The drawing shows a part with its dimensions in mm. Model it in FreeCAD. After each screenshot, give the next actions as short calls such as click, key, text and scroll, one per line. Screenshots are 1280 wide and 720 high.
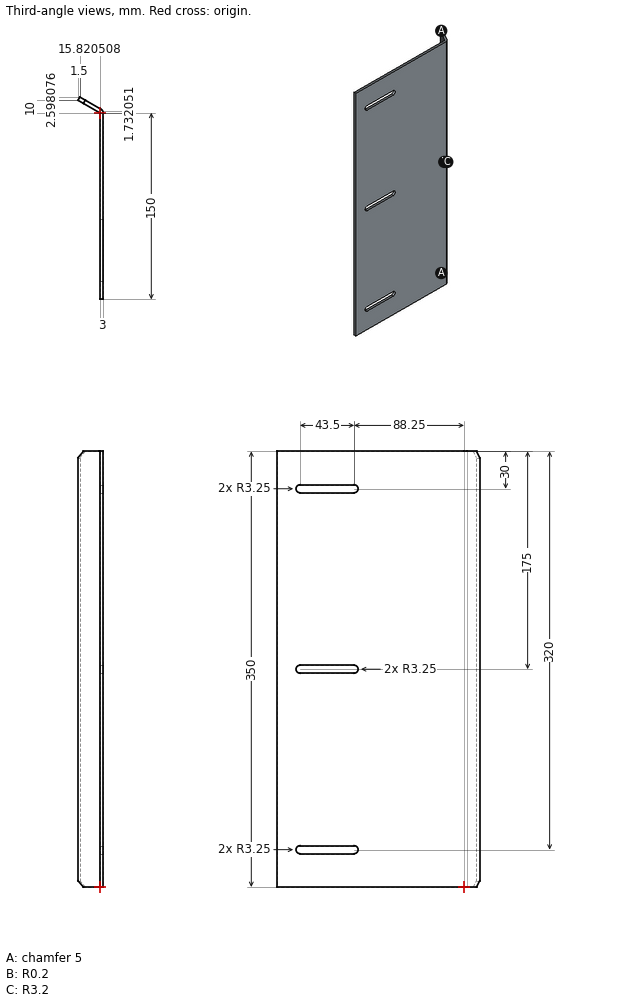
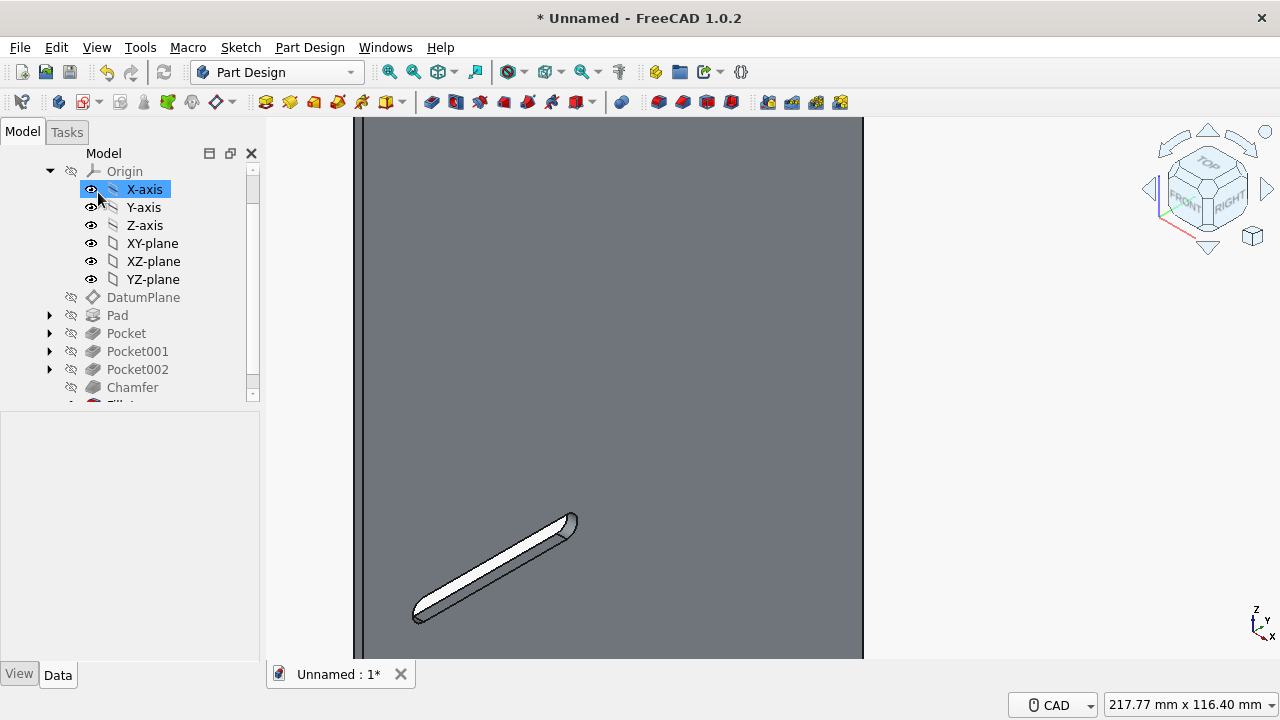
click(390, 72)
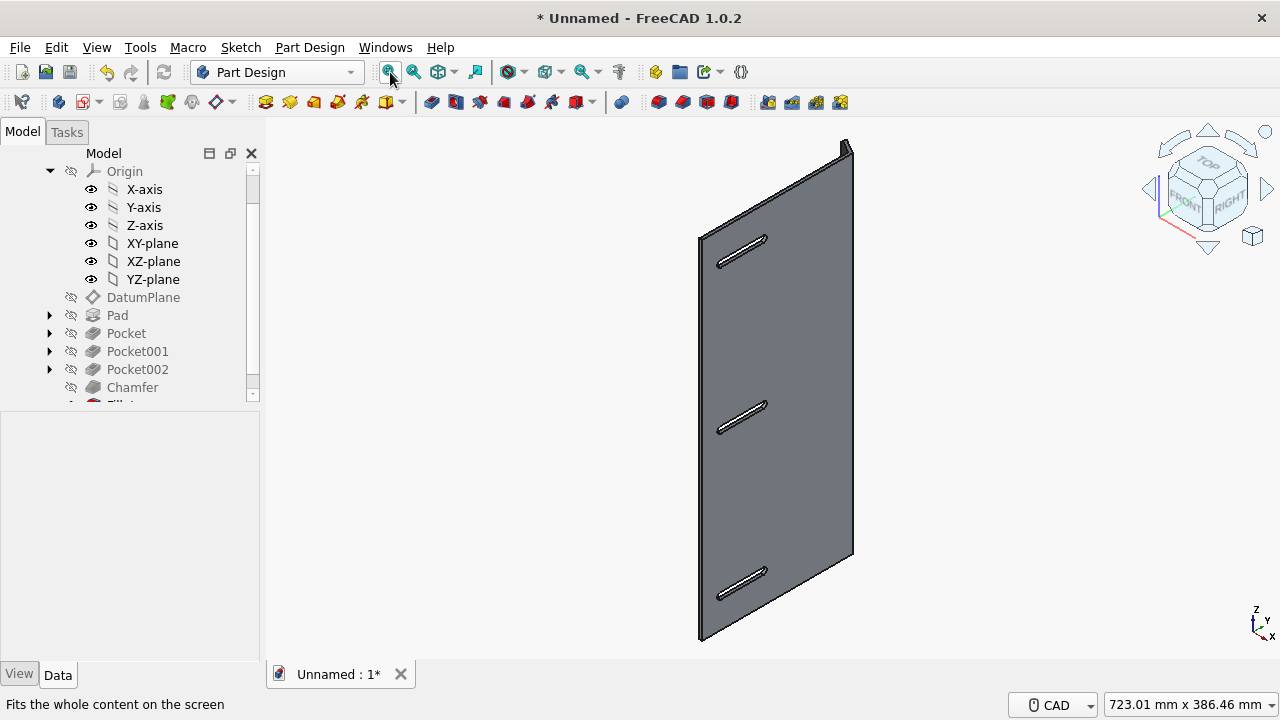
key(2)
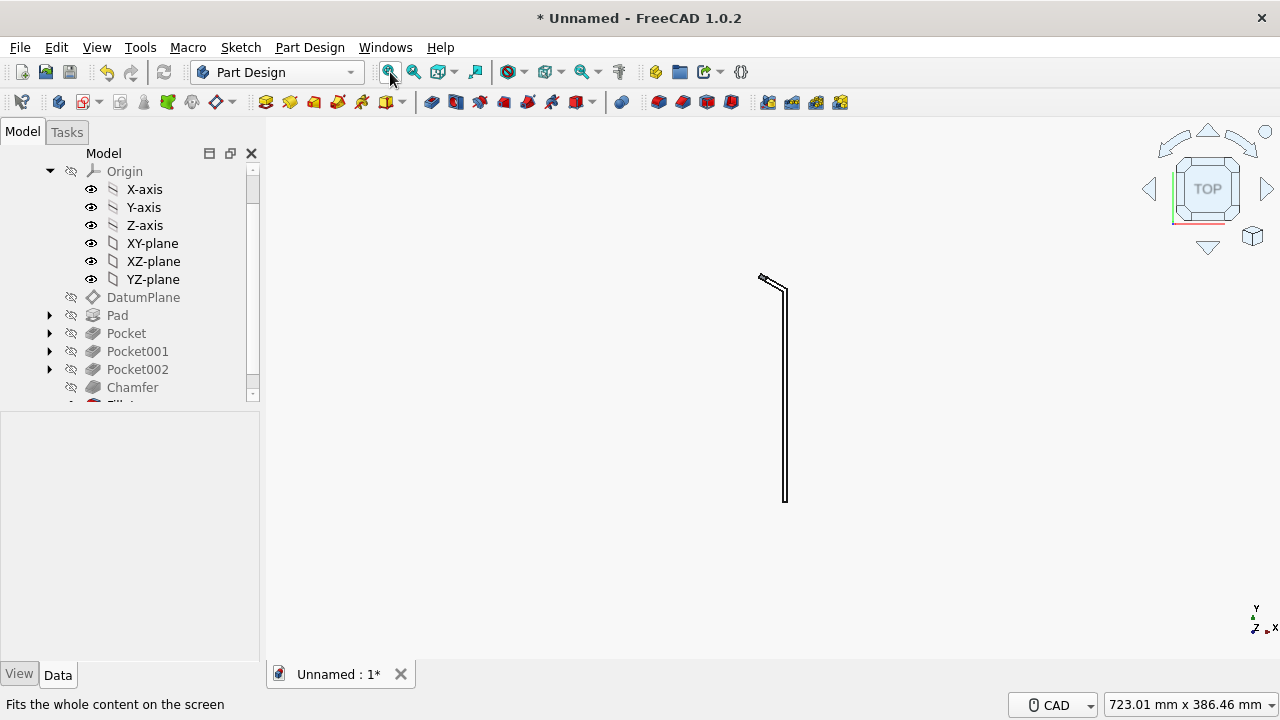
click(390, 72)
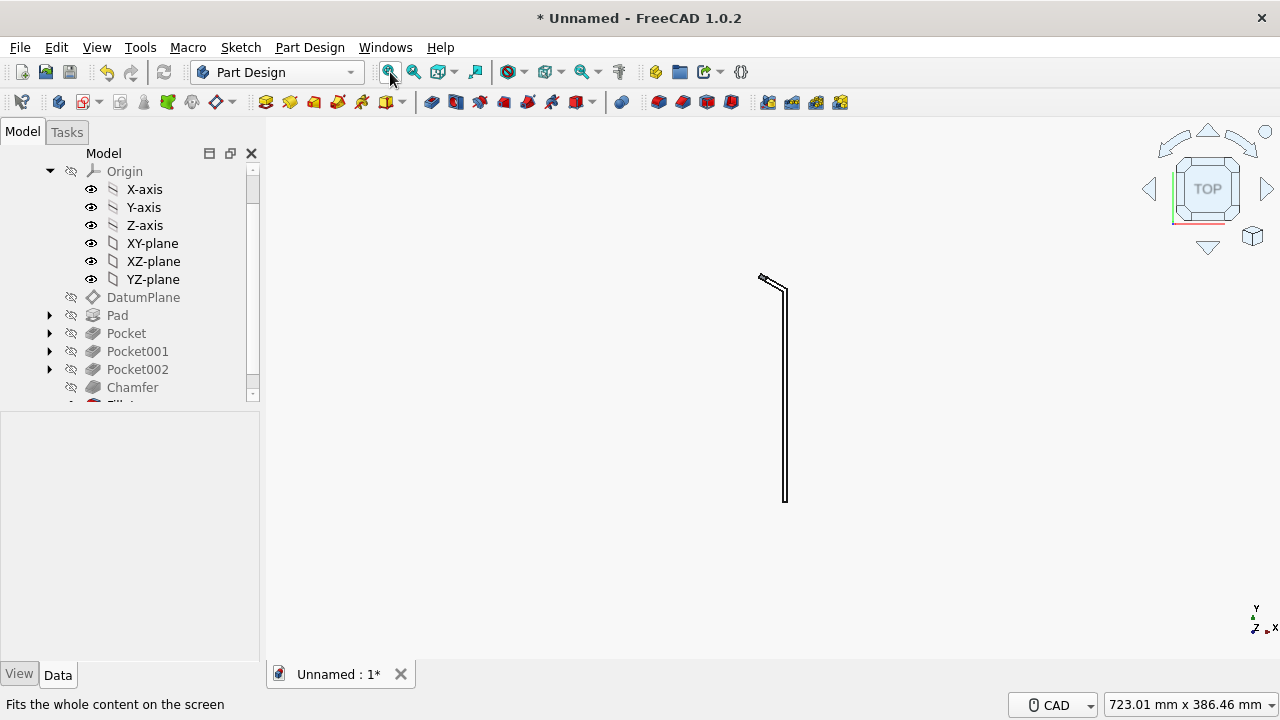
key(0)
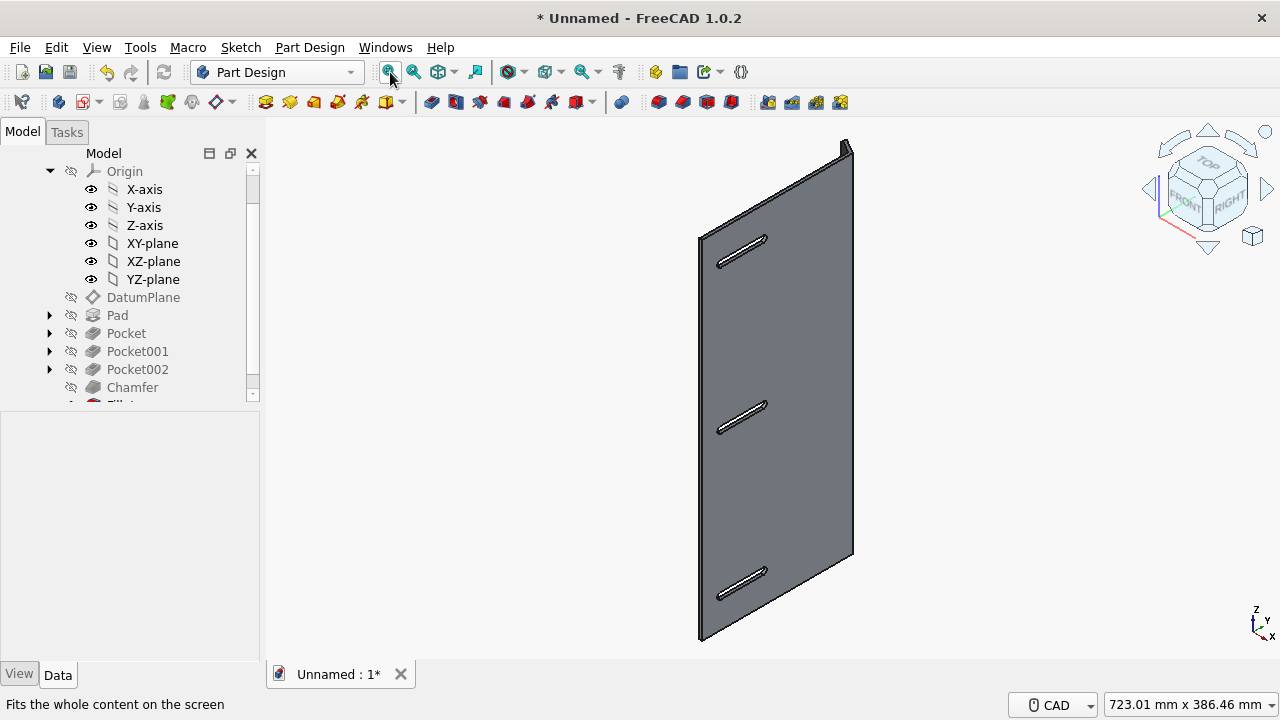
key(1)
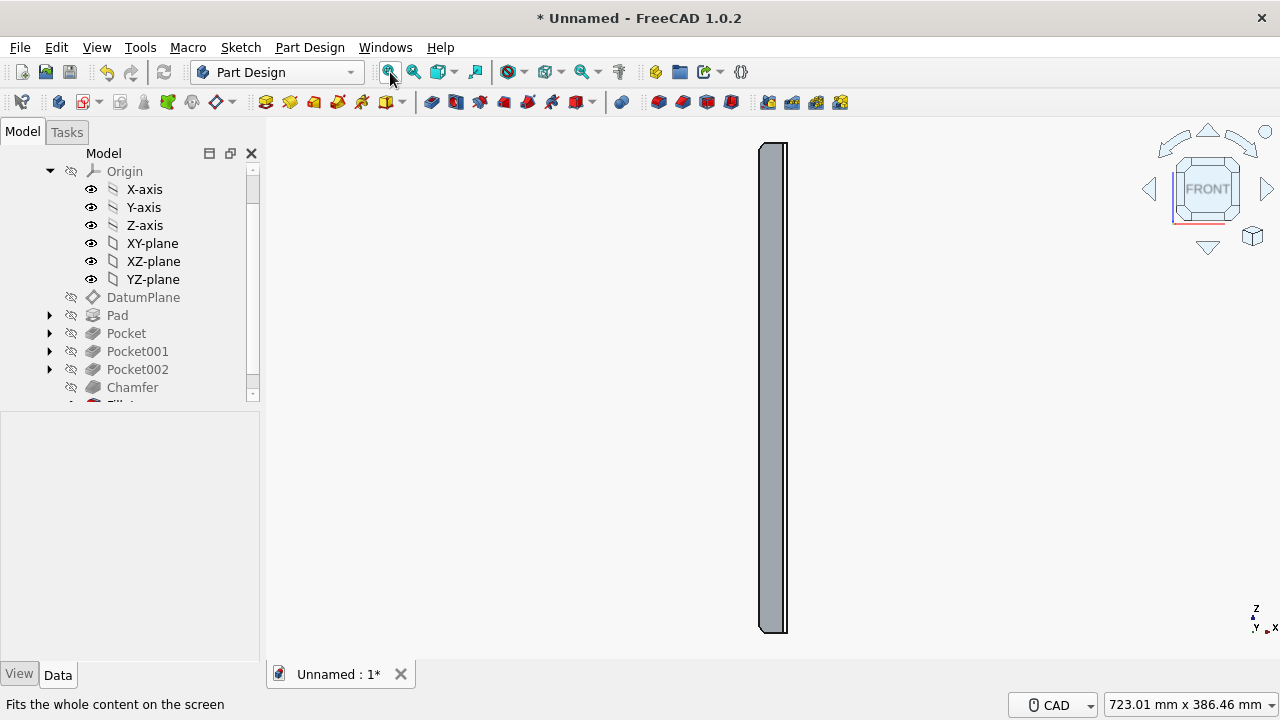
key(3)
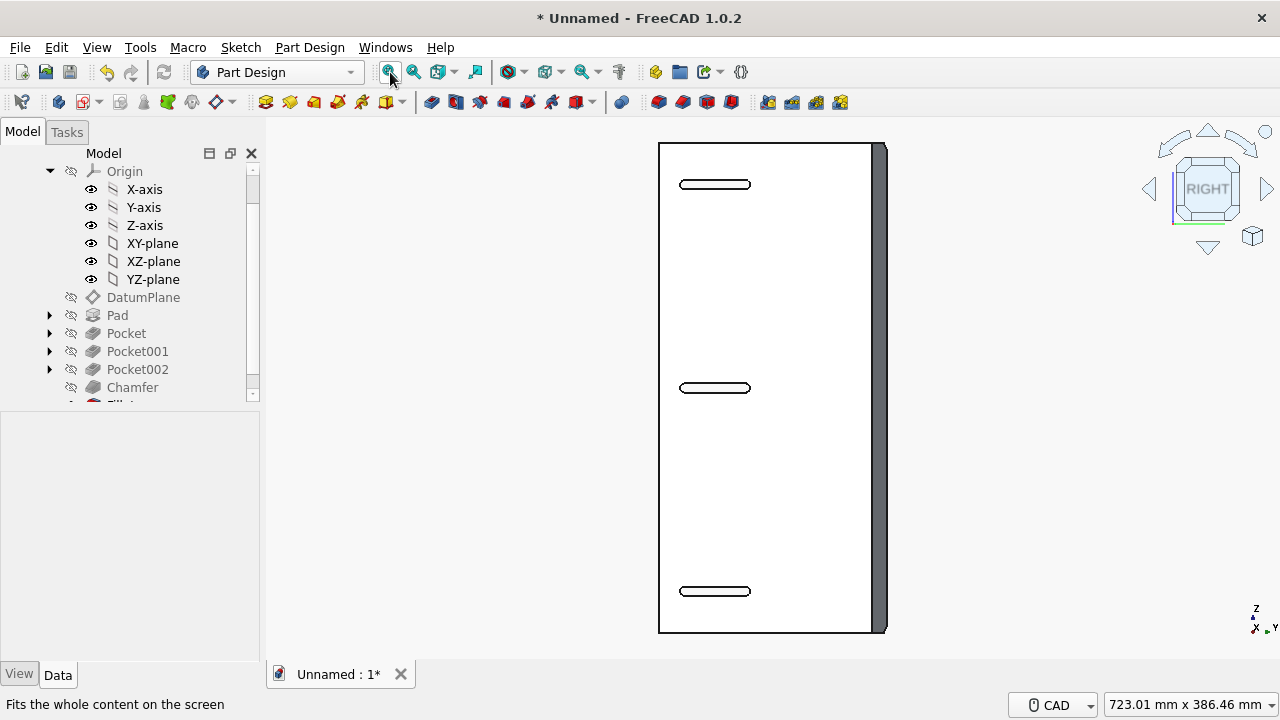
click(872, 387)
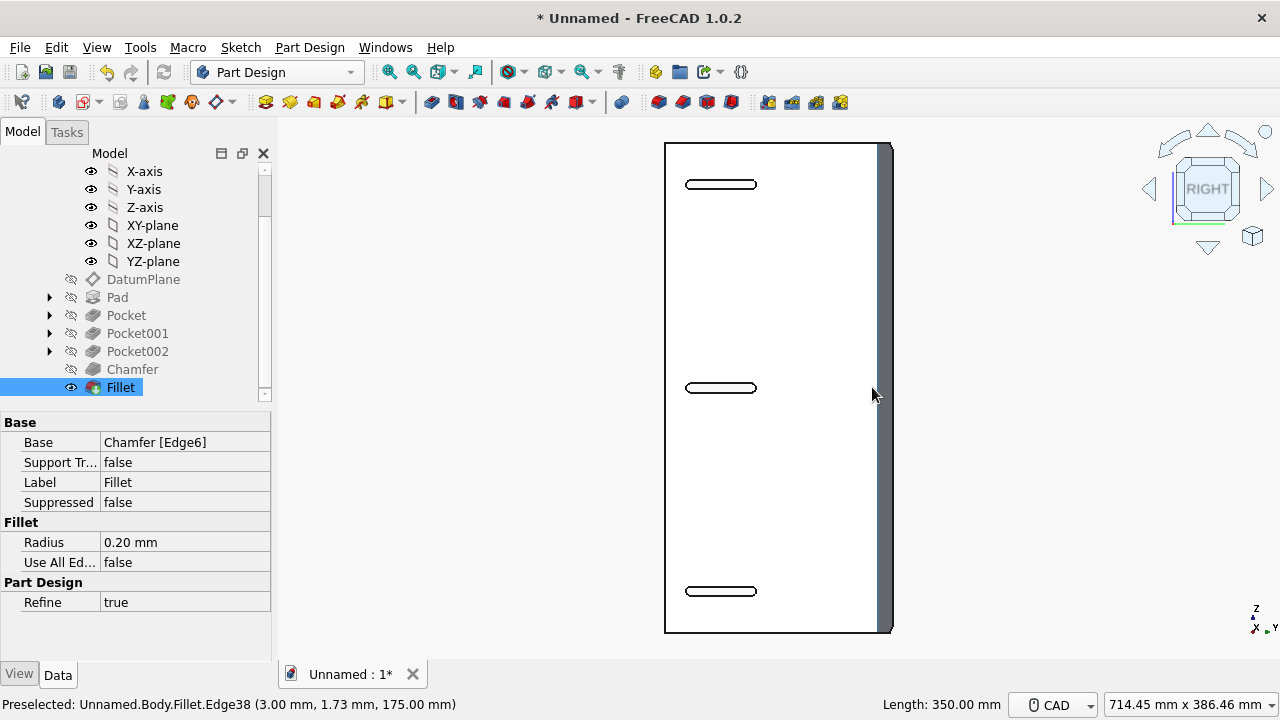
click(660, 102)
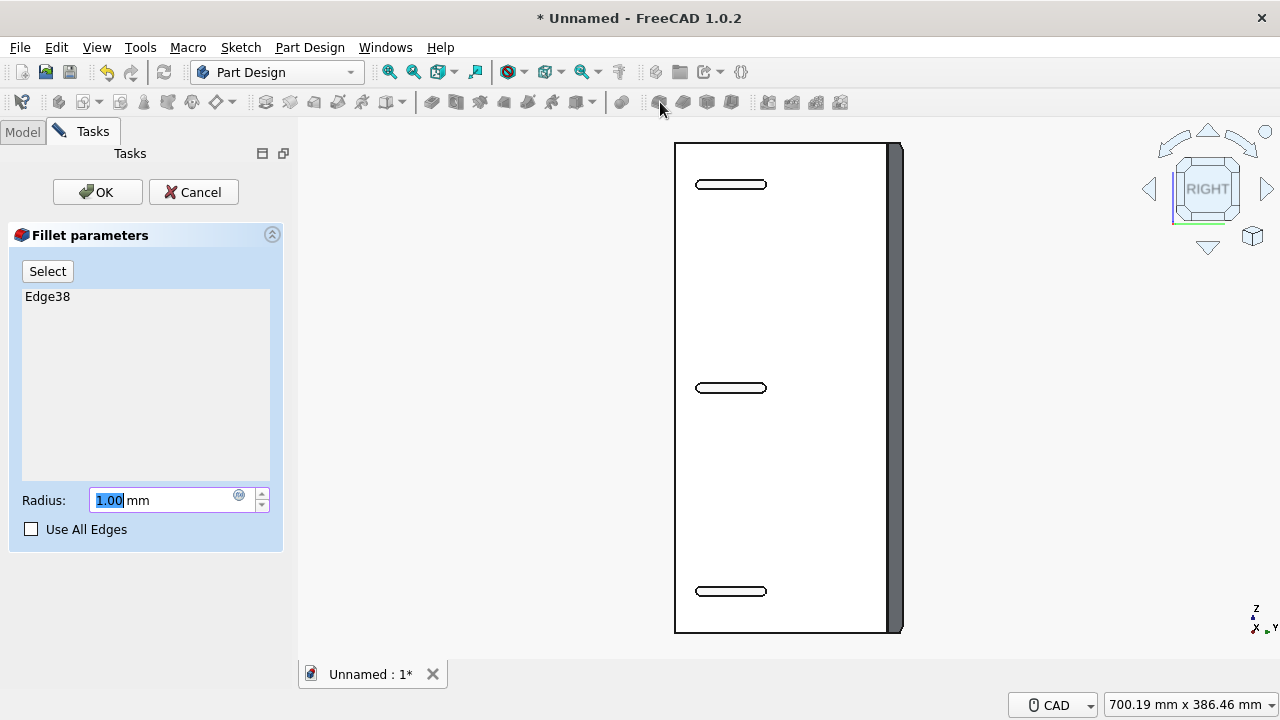
text(3.2)
key(Tab)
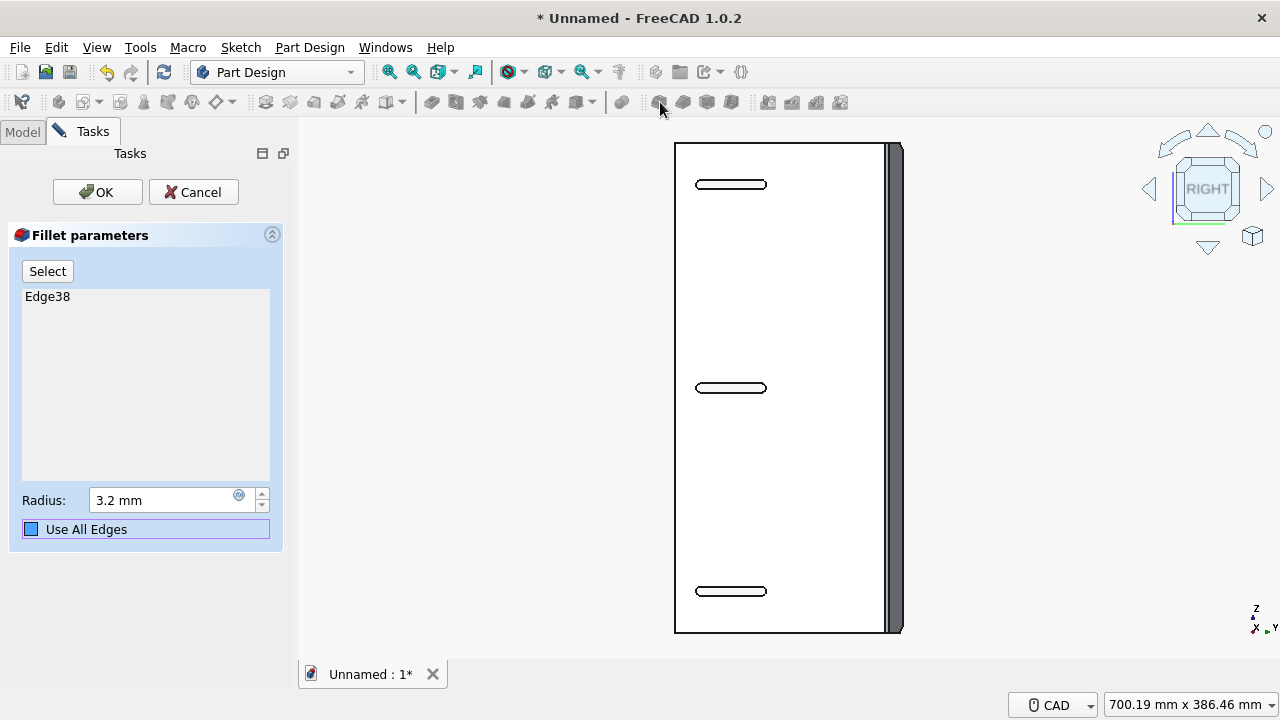
click(98, 192)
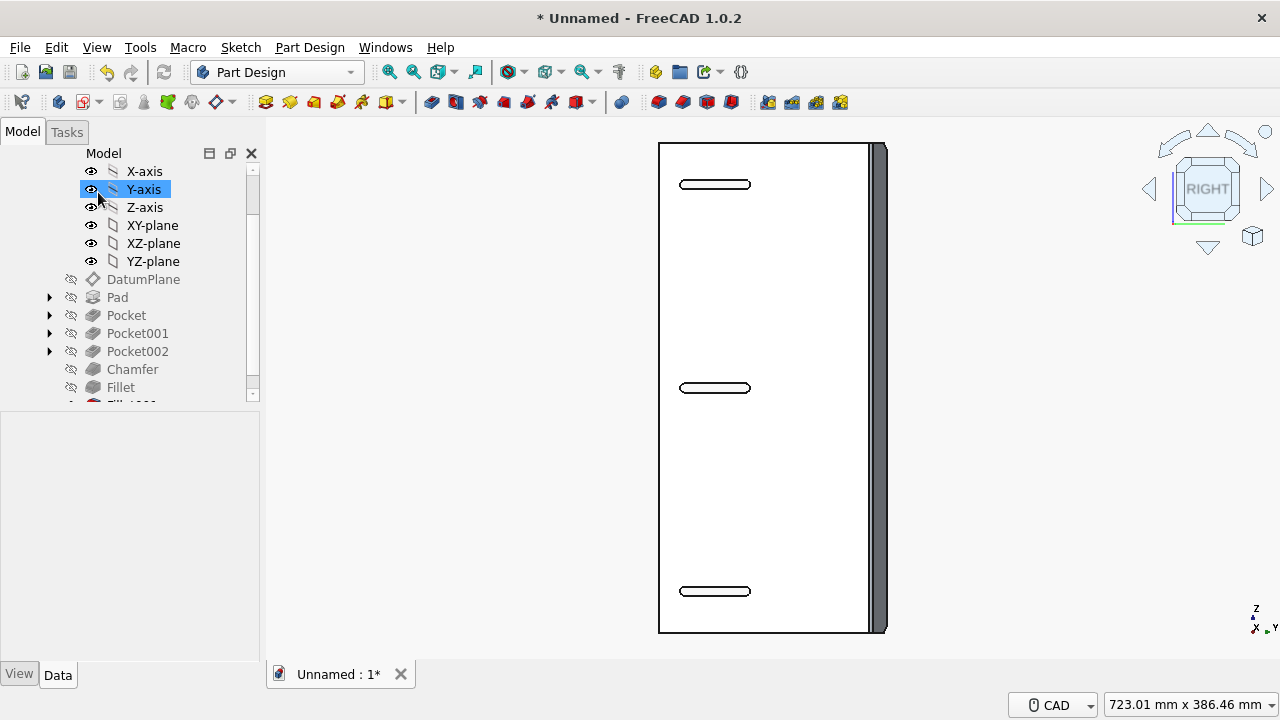
key(0)